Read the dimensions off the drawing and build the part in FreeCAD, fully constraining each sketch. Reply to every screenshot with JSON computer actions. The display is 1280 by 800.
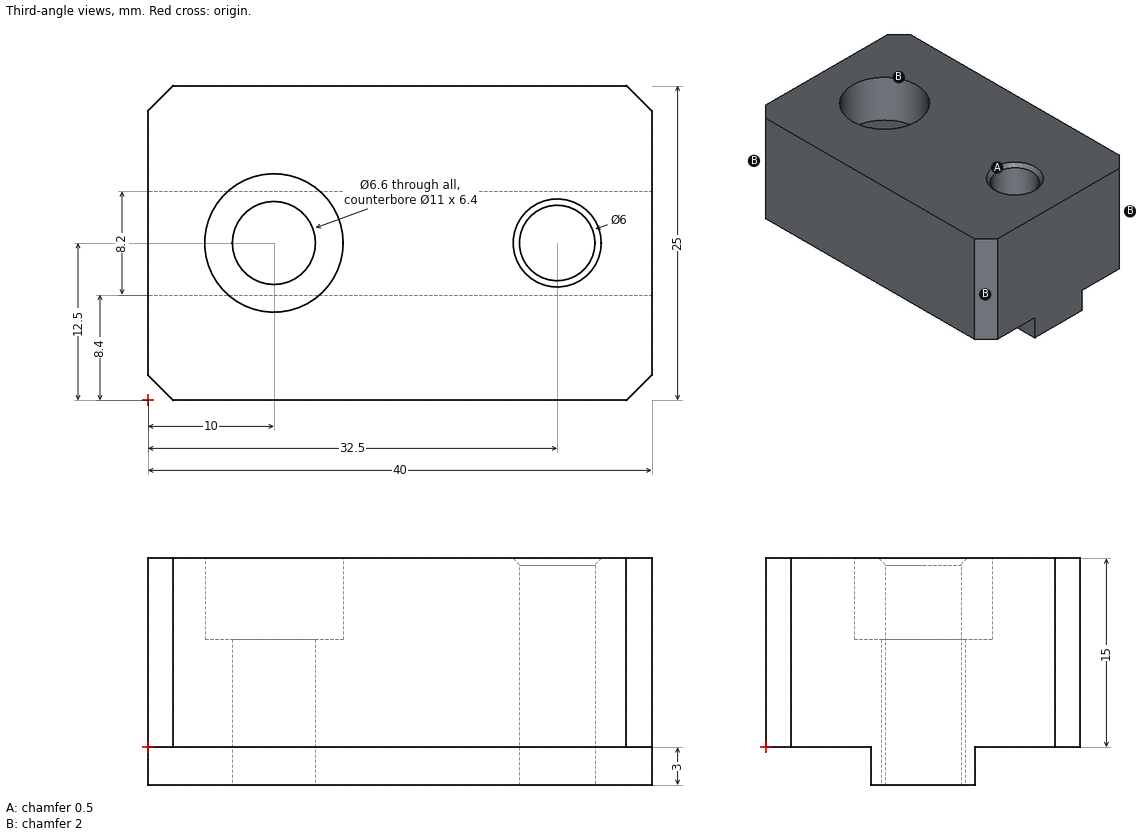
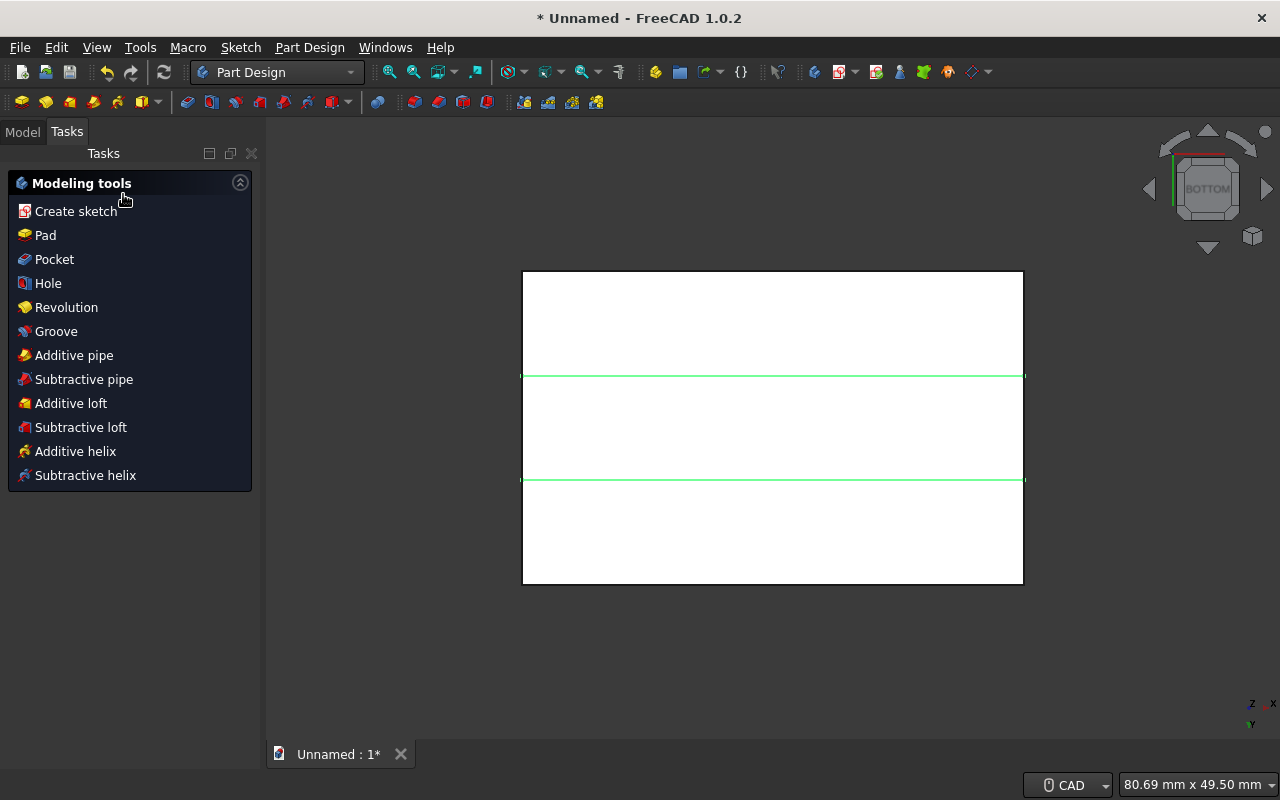
{"action": "left_click", "coordinate": [22, 102]}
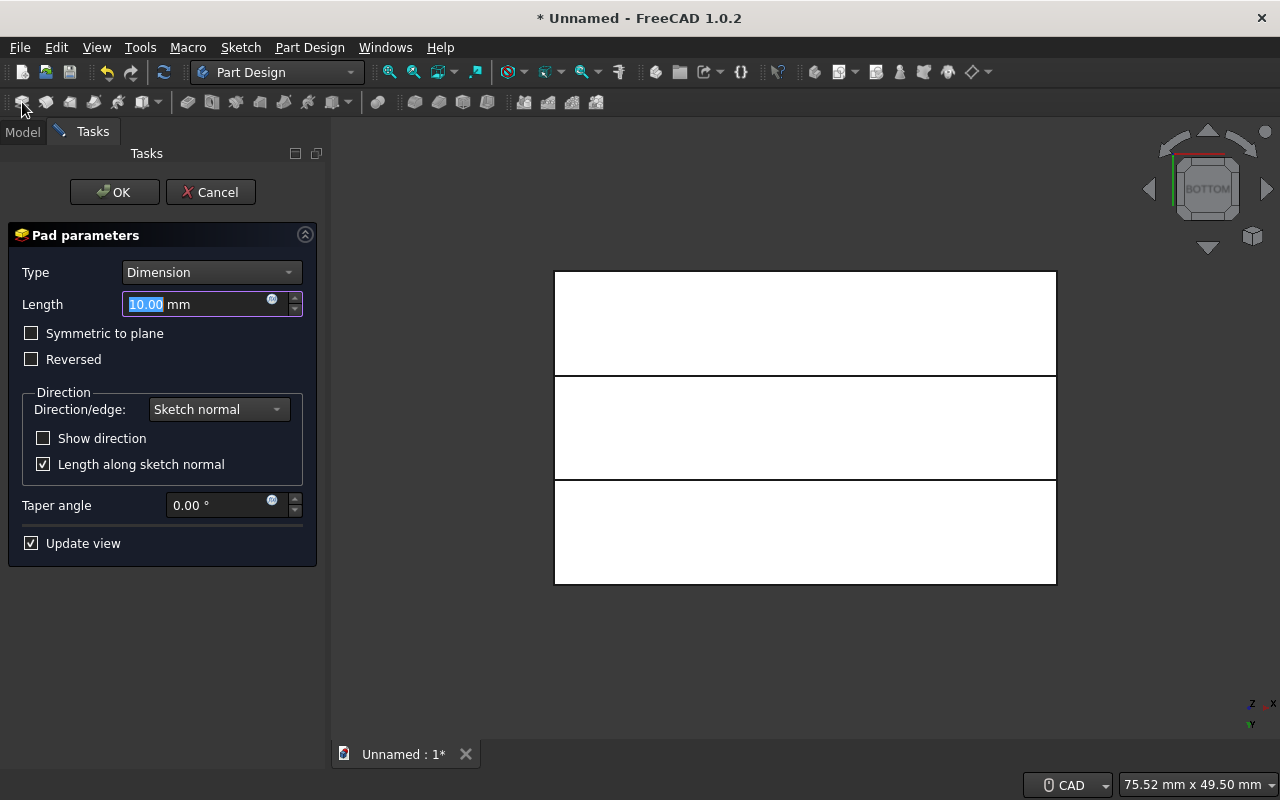
{"action": "type", "text": "3"}
{"action": "key", "text": "Tab"}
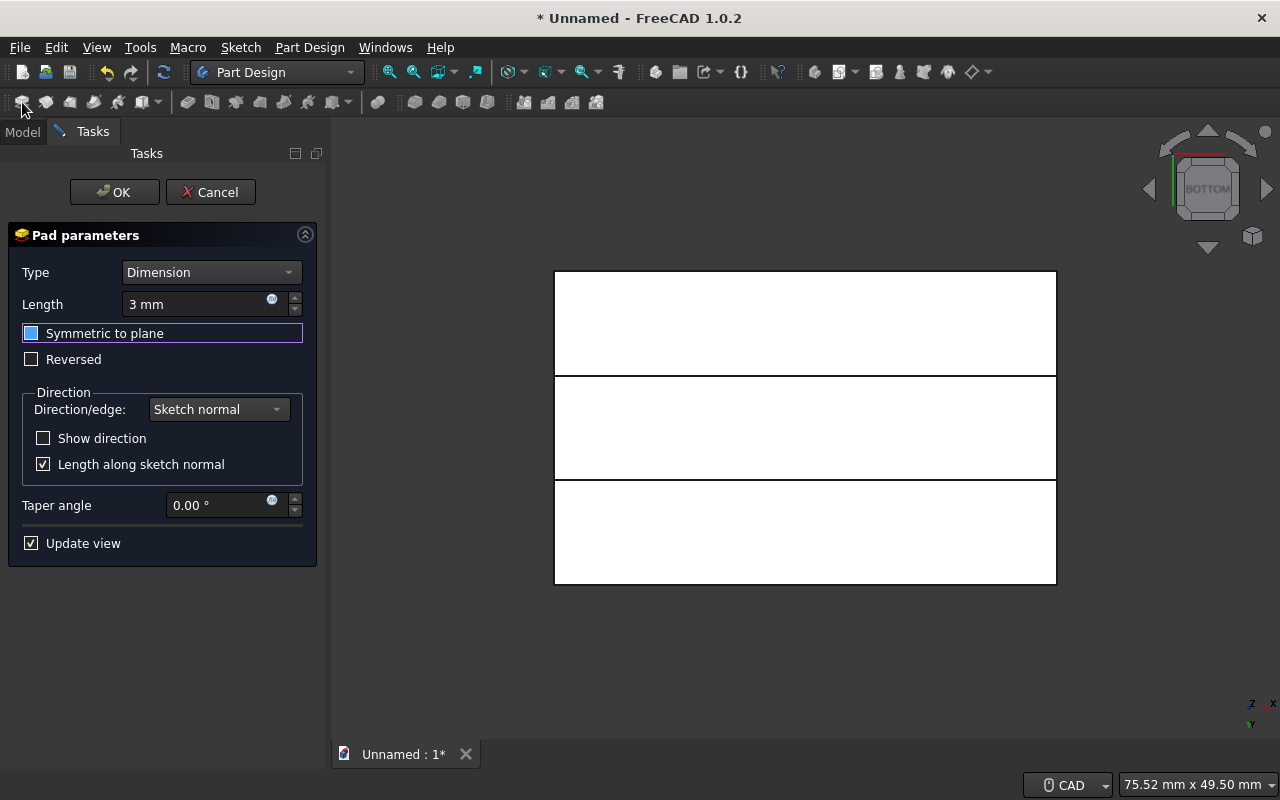
{"action": "left_click", "coordinate": [115, 192]}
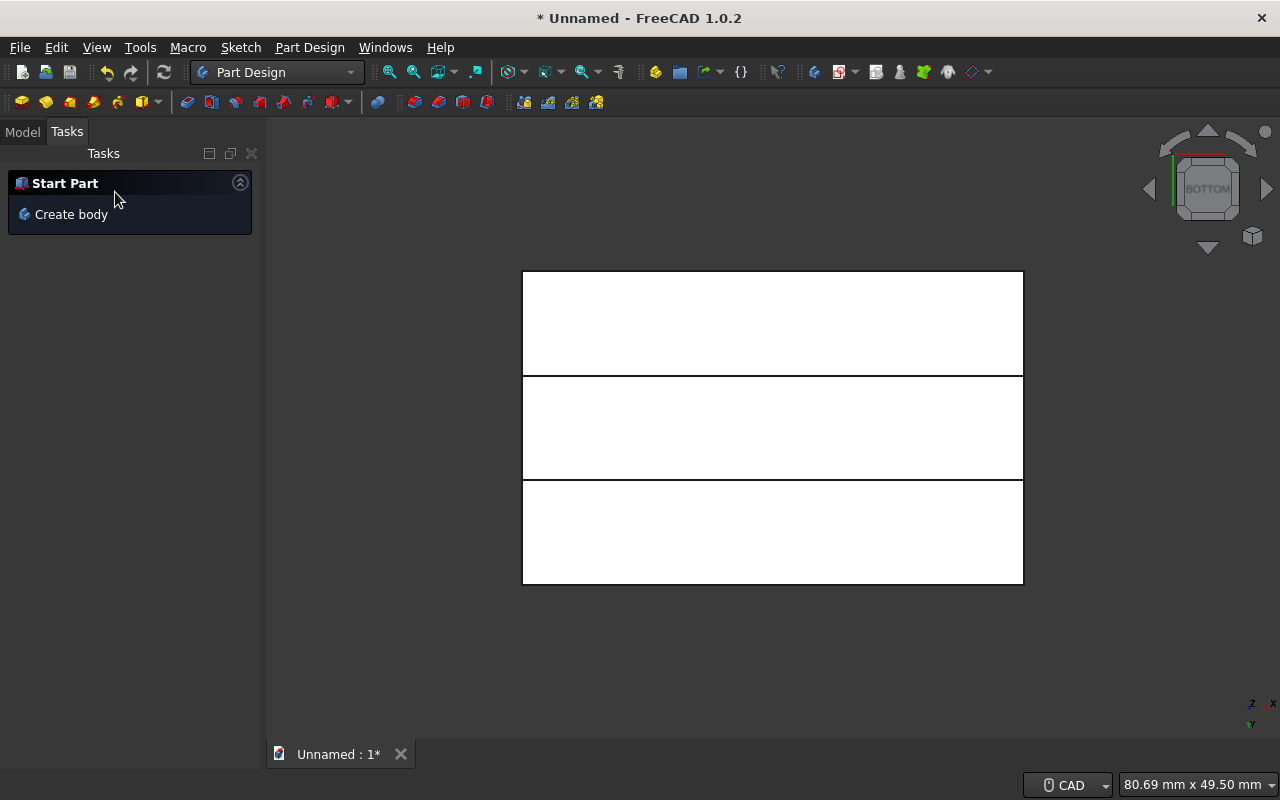
{"action": "key", "text": "0"}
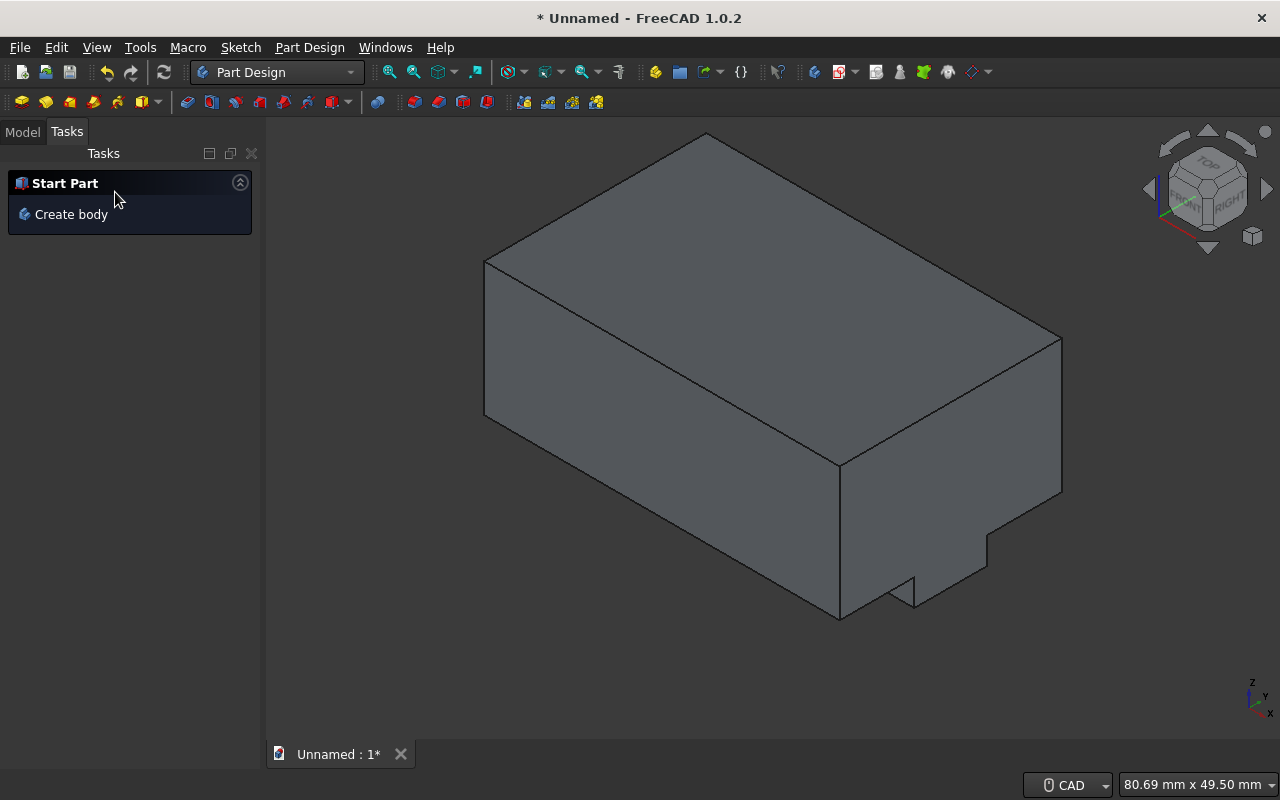
{"action": "left_click", "coordinate": [824, 328]}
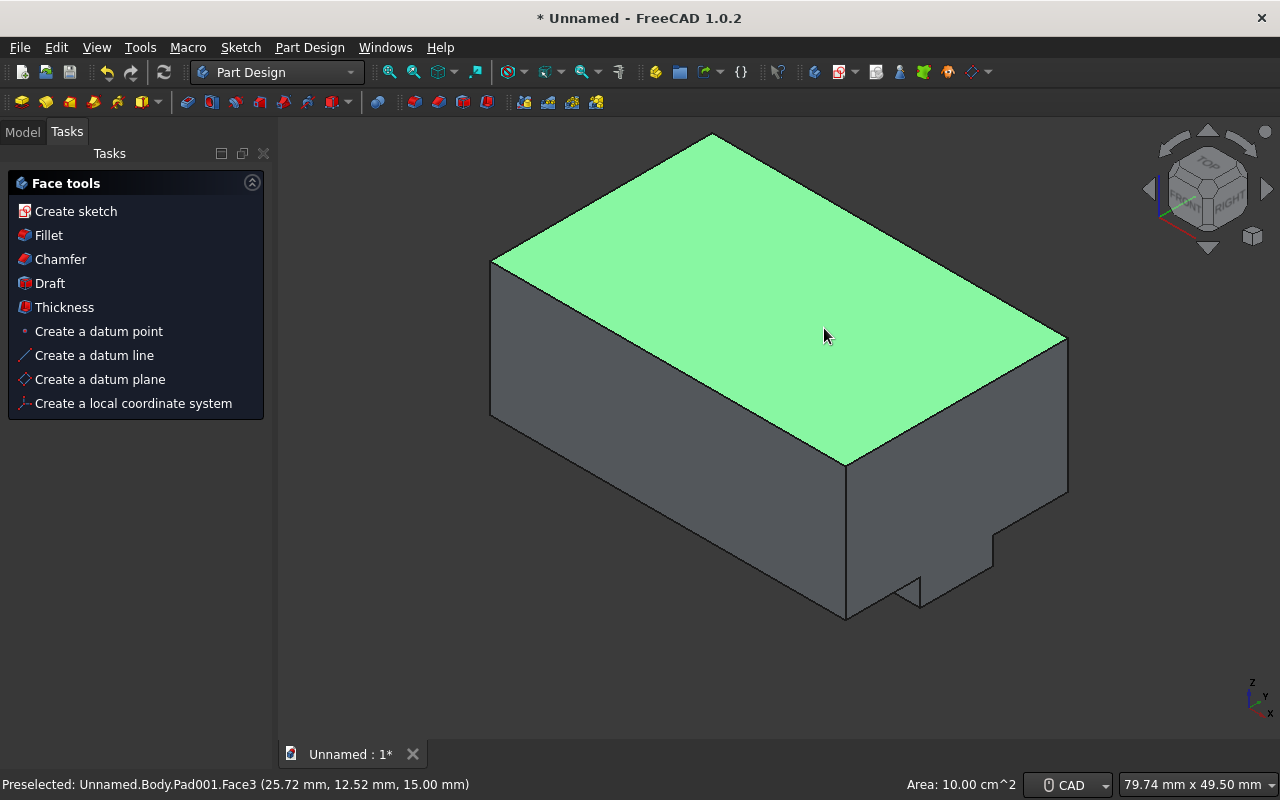
{"action": "left_click", "coordinate": [840, 72]}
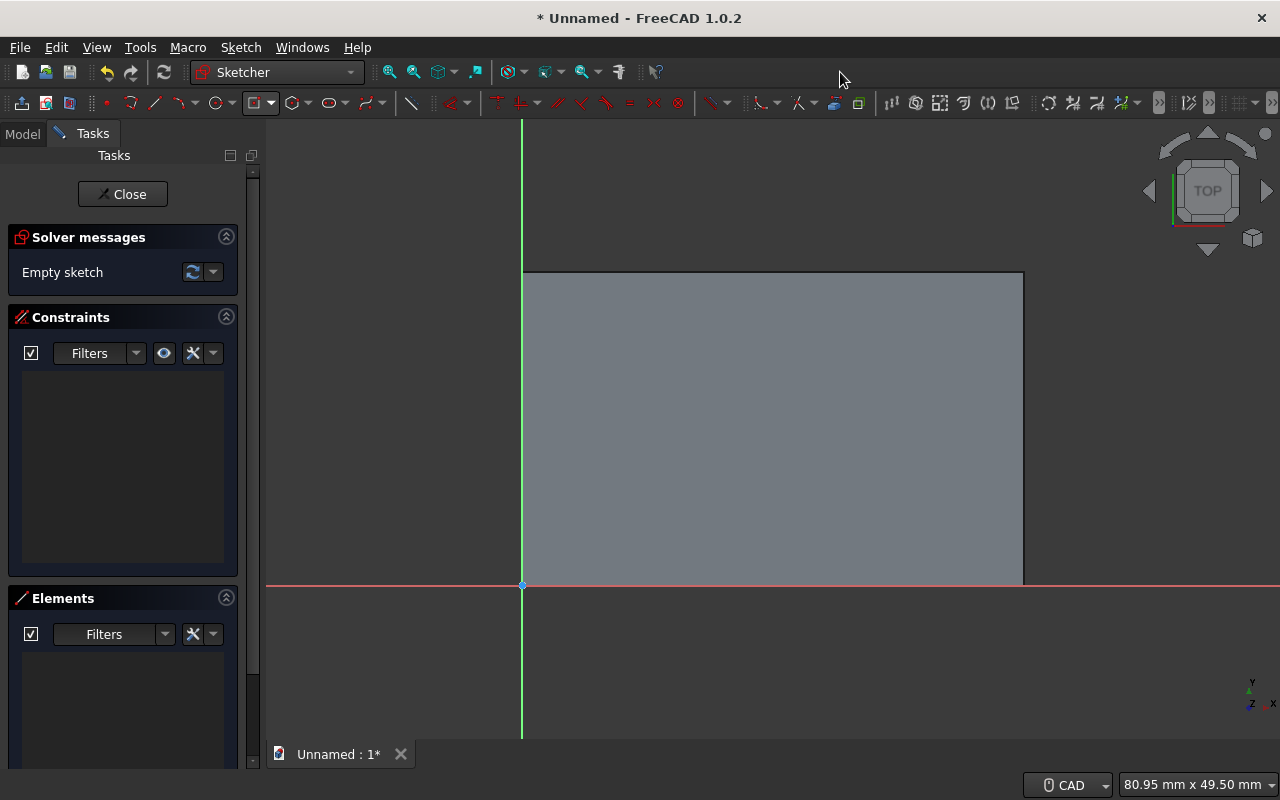
{"action": "scroll", "coordinate": [486, 557], "scroll_direction": "up", "scroll_amount": 3}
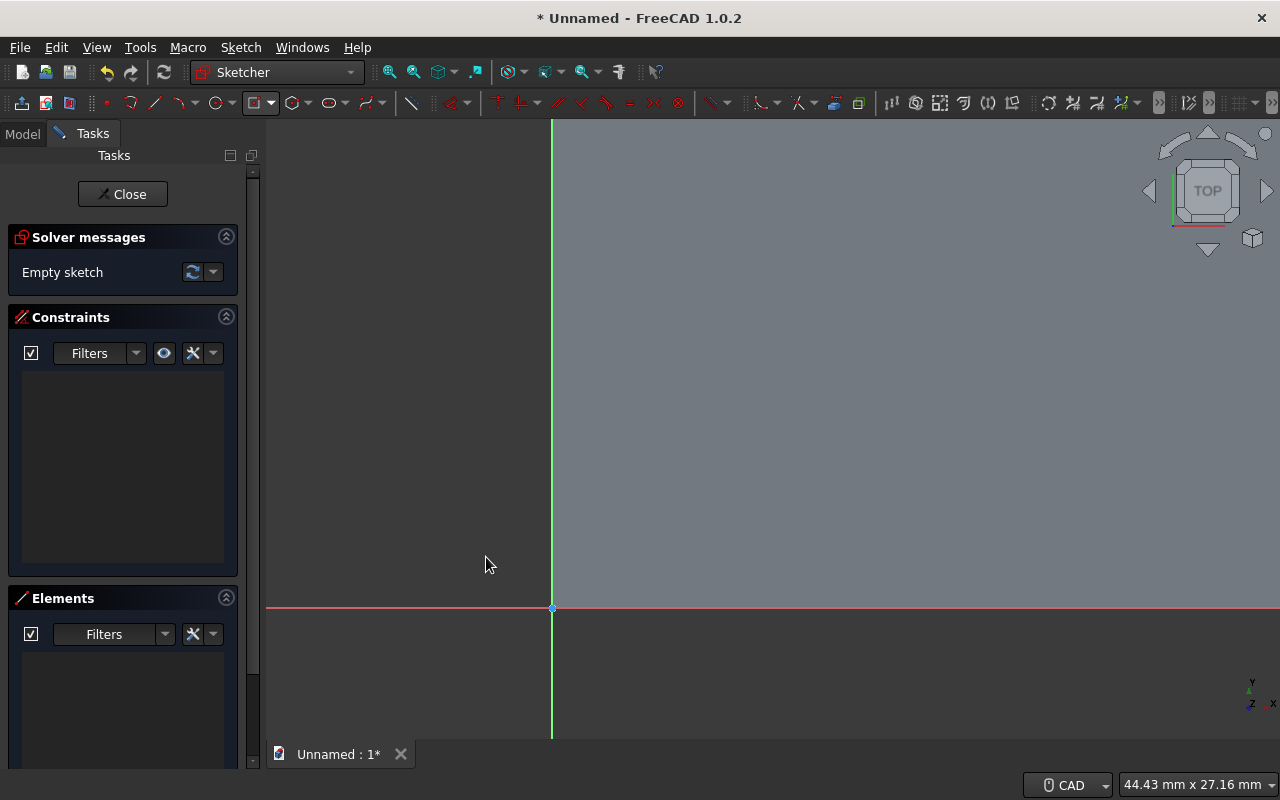
{"action": "left_click", "coordinate": [216, 104]}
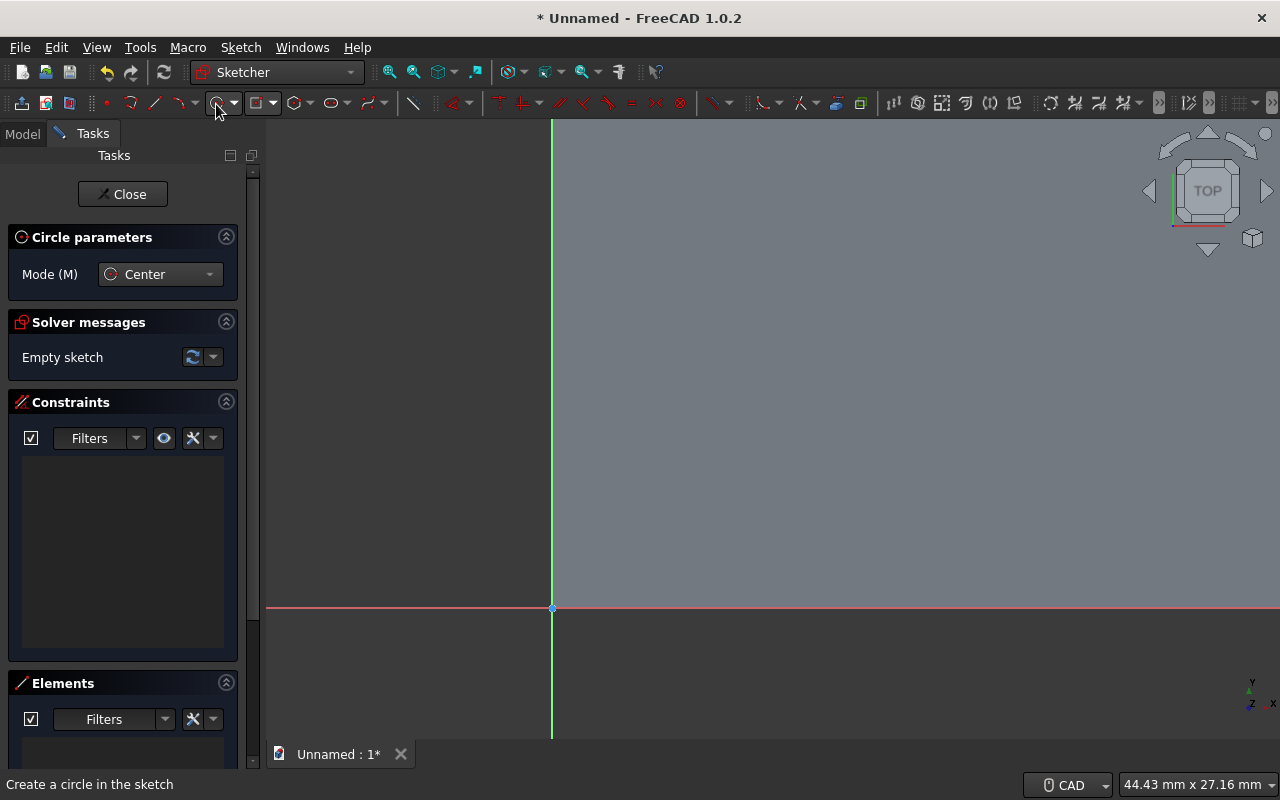
{"action": "left_click", "coordinate": [781, 323]}
{"action": "left_click", "coordinate": [834, 270]}
{"action": "key", "text": "Escape"}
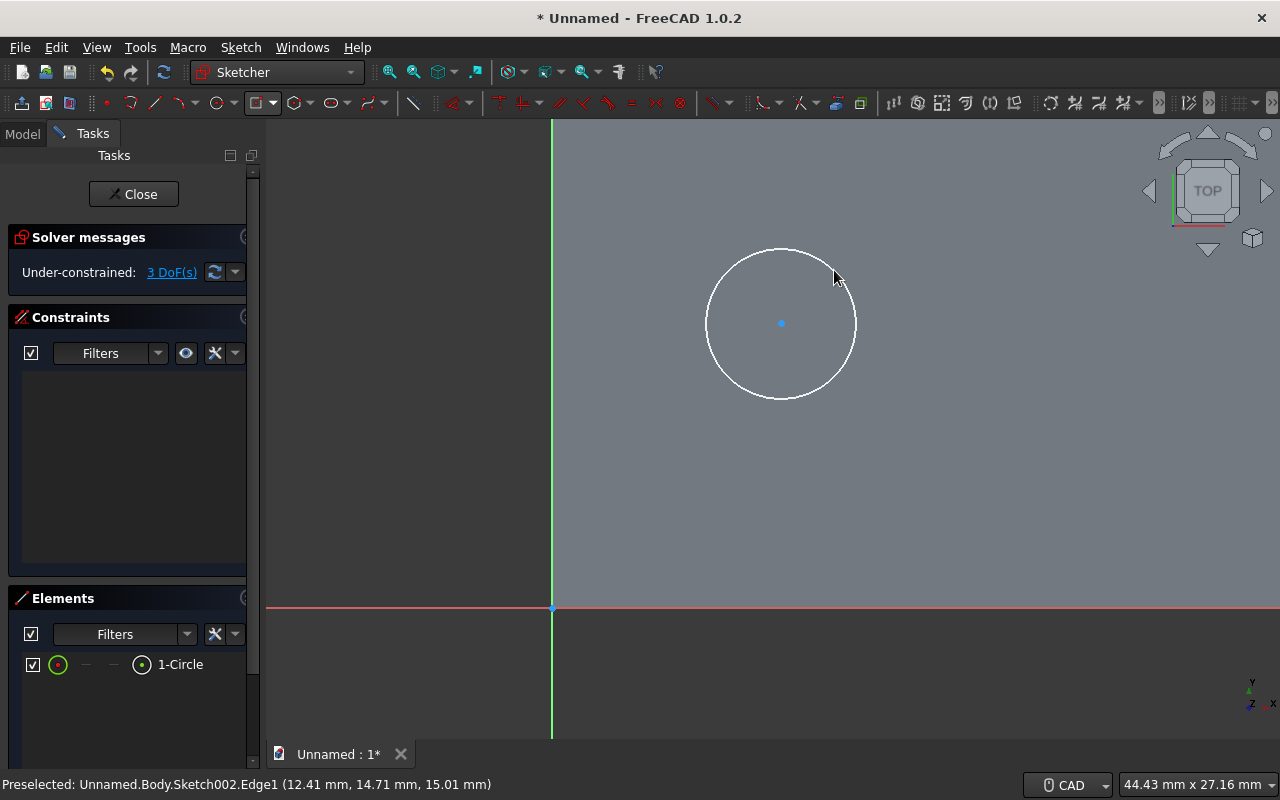
{"action": "left_click", "coordinate": [452, 104]}